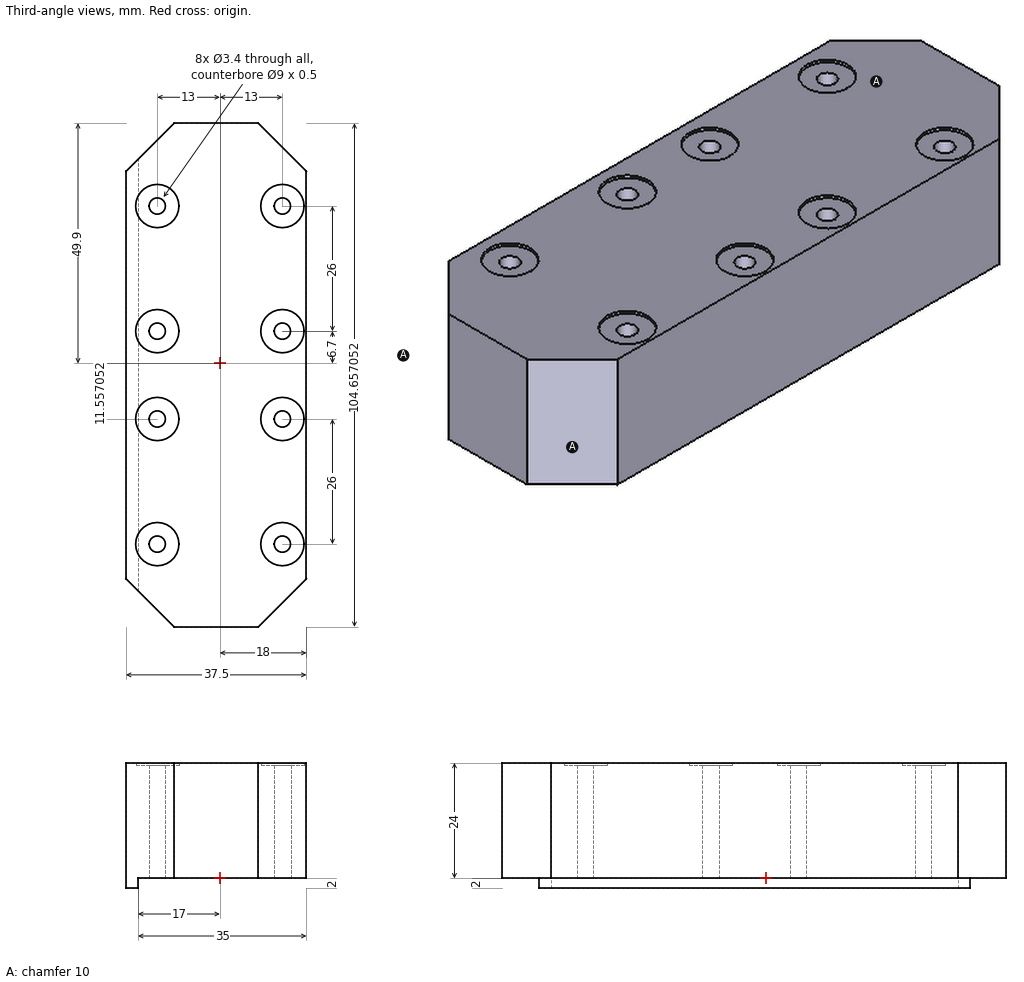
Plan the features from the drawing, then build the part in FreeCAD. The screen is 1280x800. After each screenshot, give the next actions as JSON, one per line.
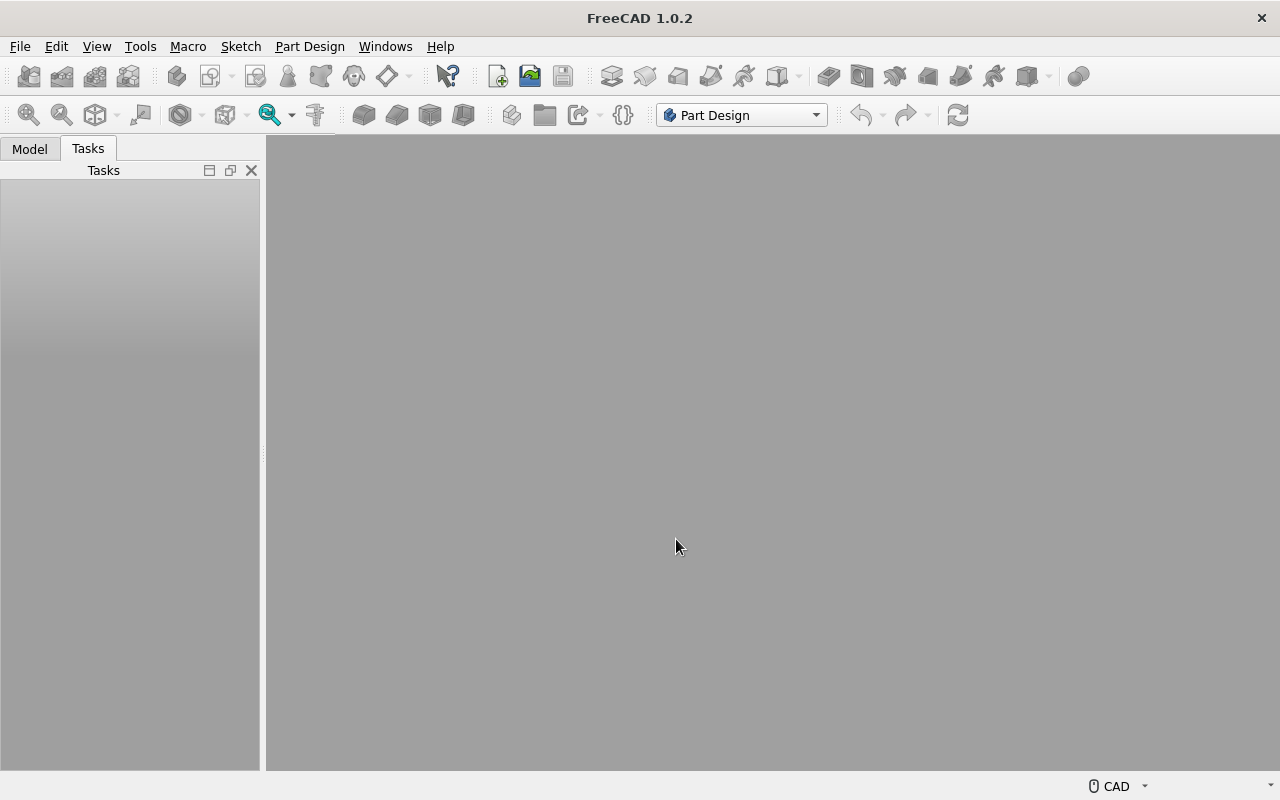
{"action": "left_click", "coordinate": [497, 76]}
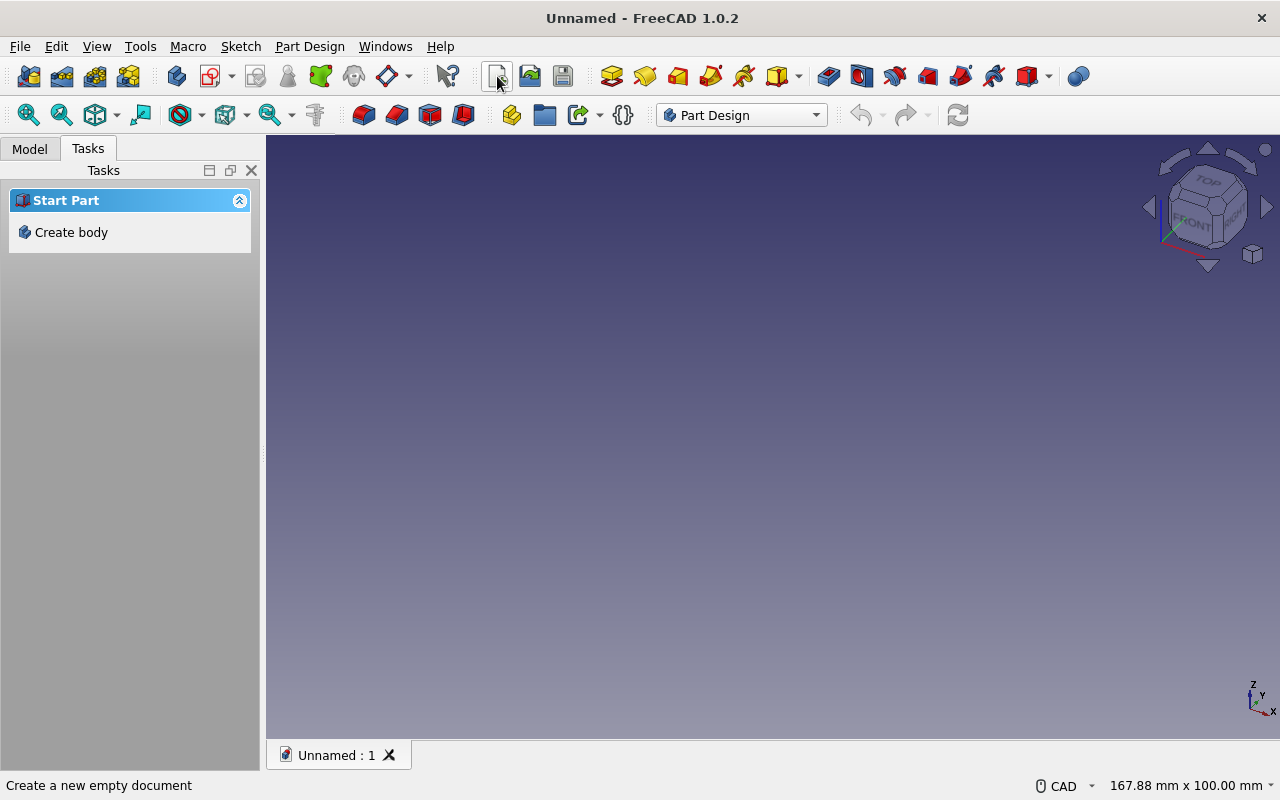
{"action": "left_click", "coordinate": [210, 76]}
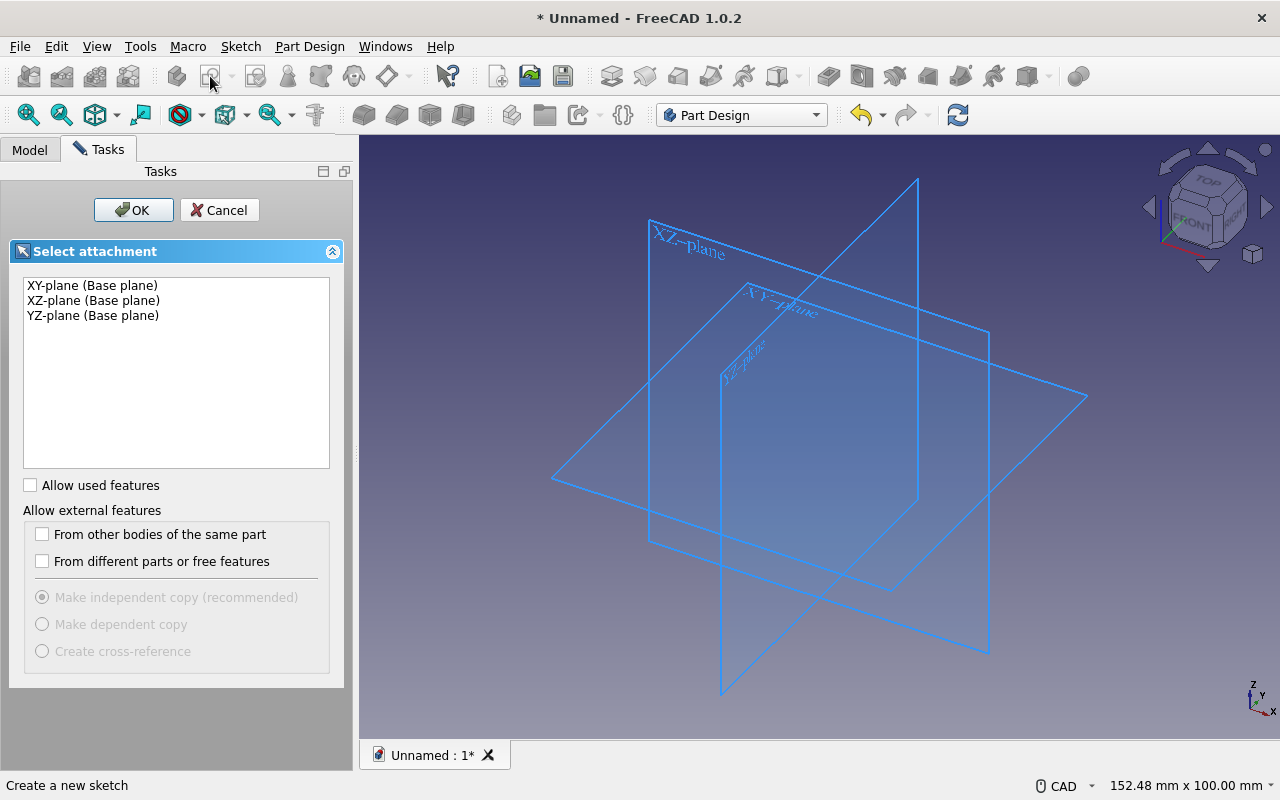
{"action": "left_click", "coordinate": [84, 286]}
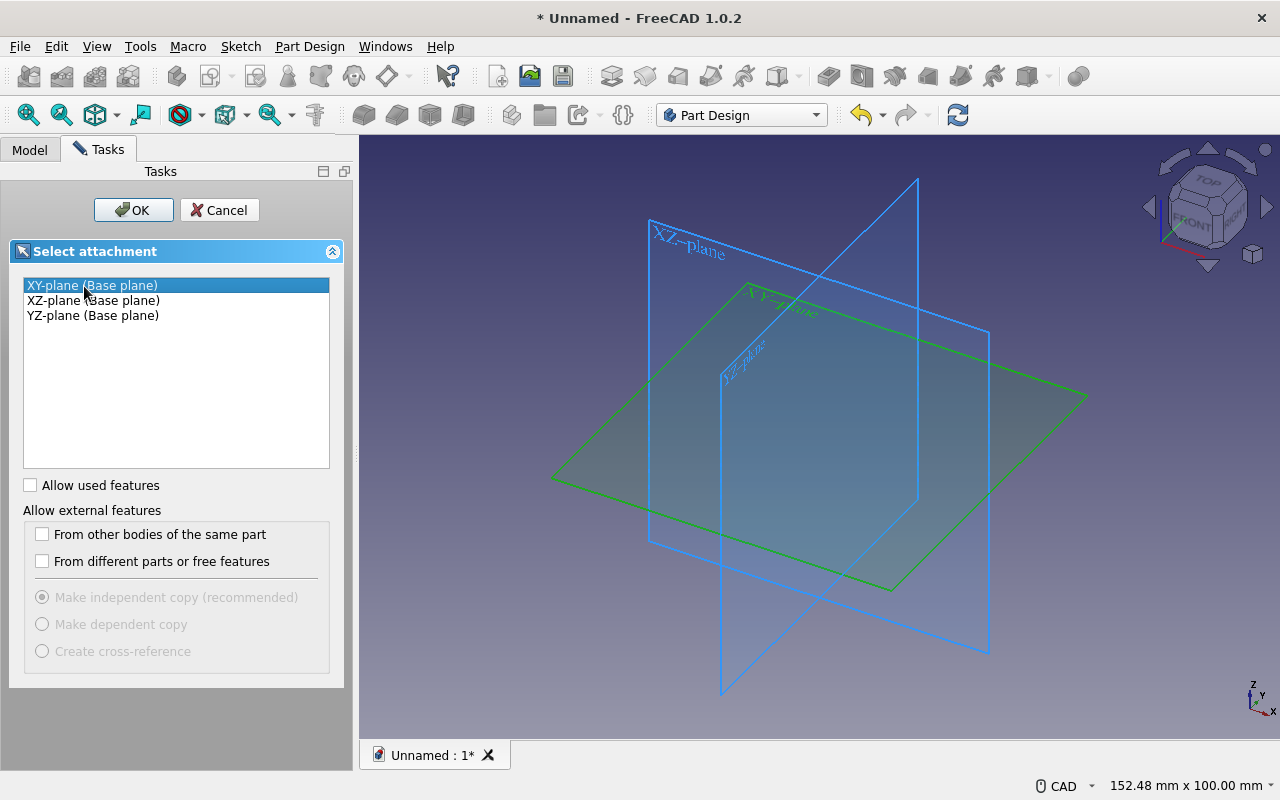
{"action": "left_click", "coordinate": [134, 210]}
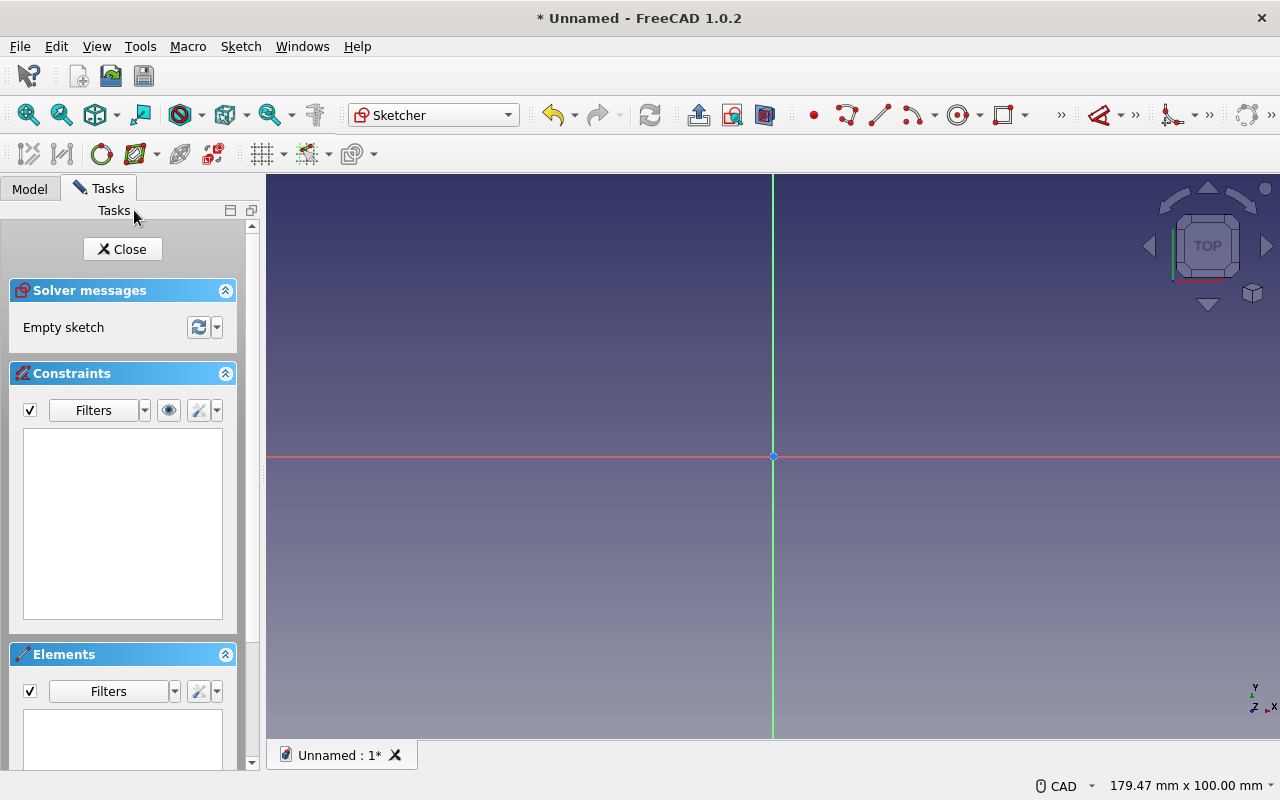
{"action": "scroll", "coordinate": [574, 429], "scroll_direction": "down", "scroll_amount": 2}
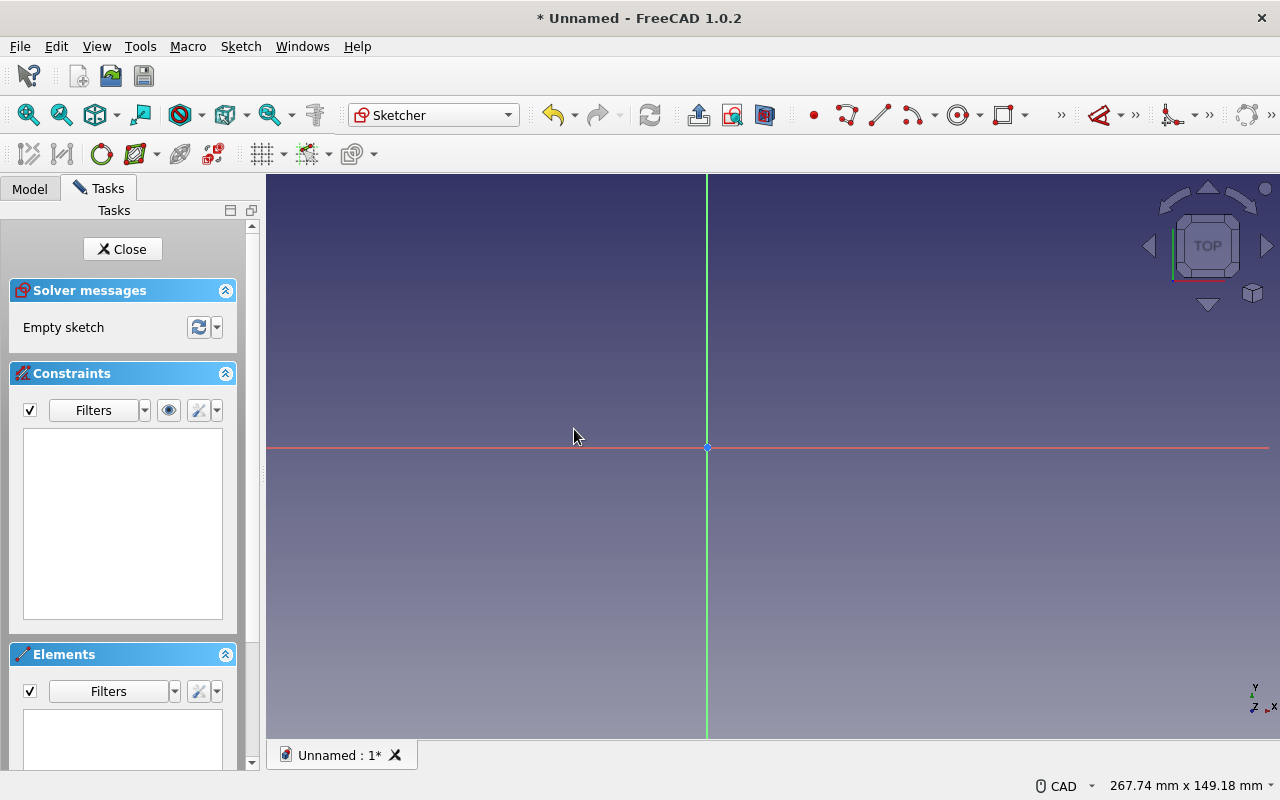
{"action": "left_click", "coordinate": [1002, 116]}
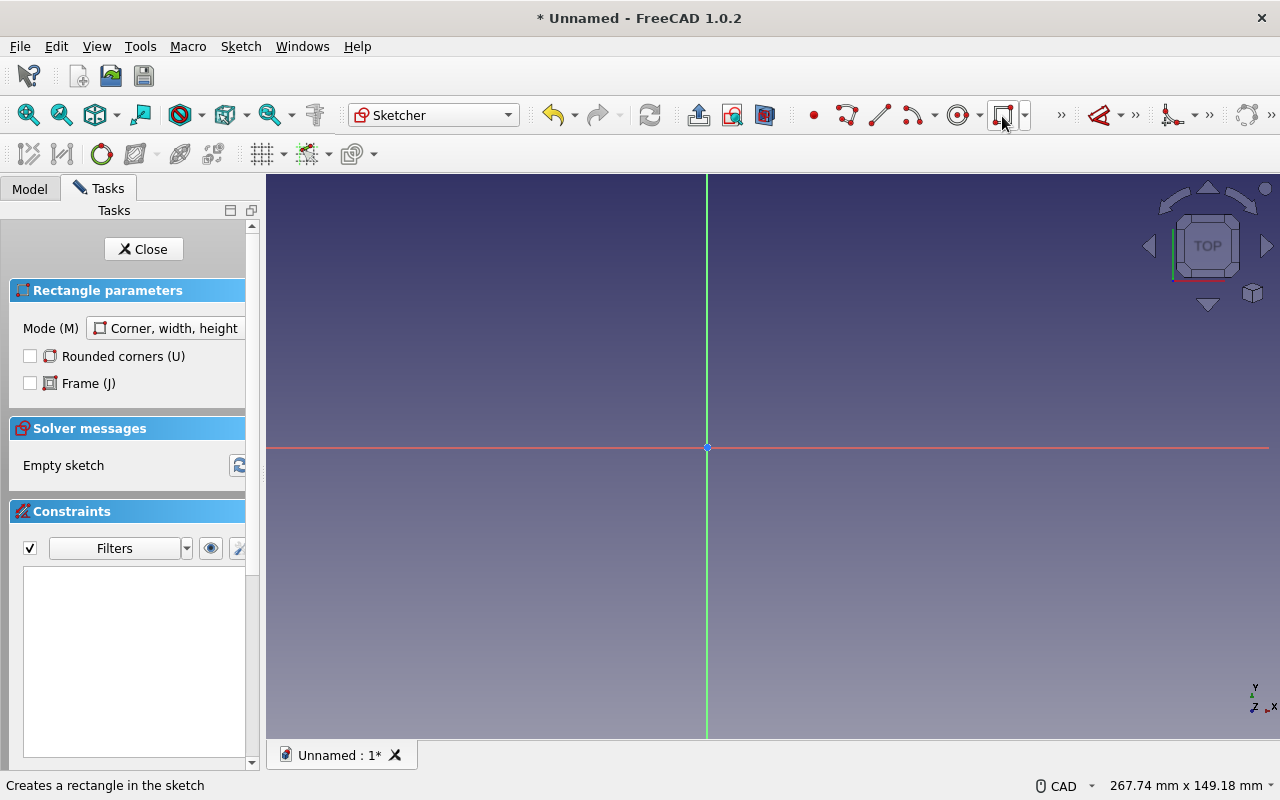
{"action": "left_click", "coordinate": [634, 259]}
{"action": "mouse_move", "coordinate": [776, 655]}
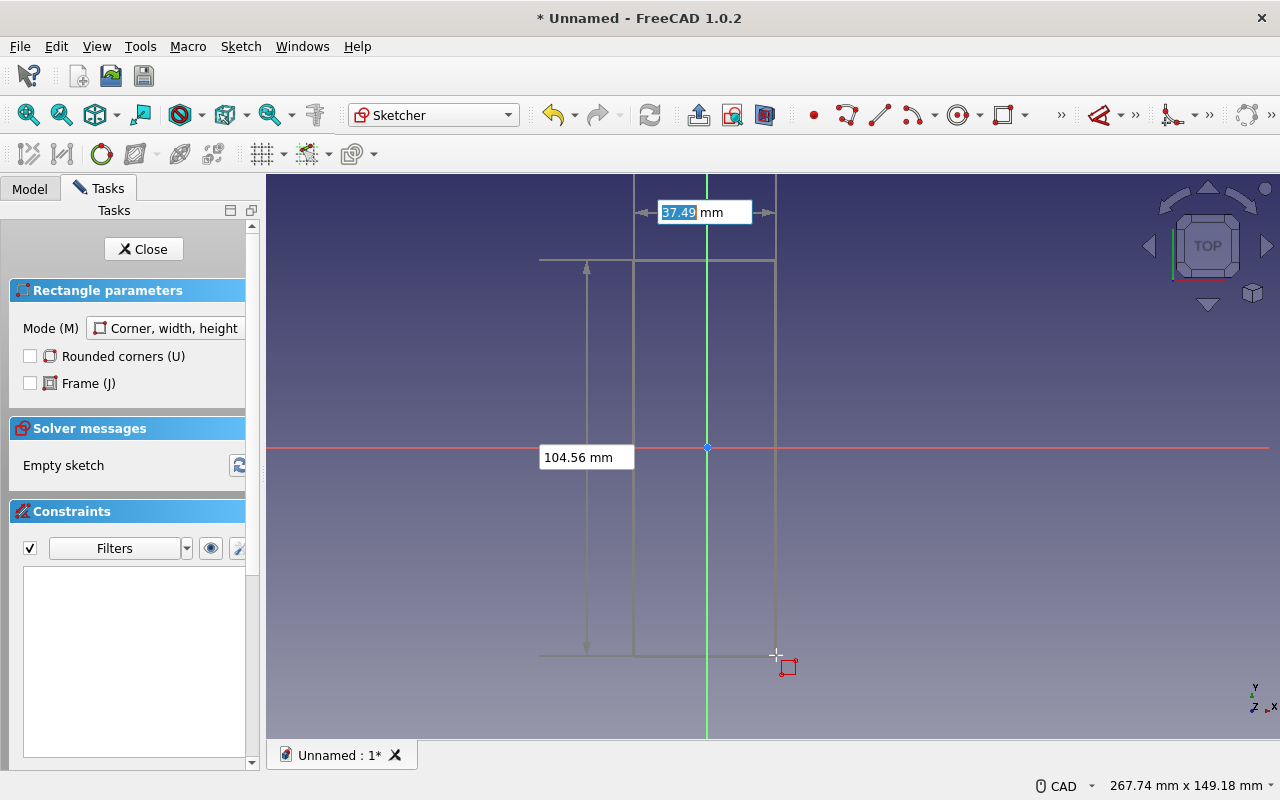
{"action": "type", "text": "37.5"}
{"action": "key", "text": "Tab"}
{"action": "type", "text": "104.657052"}
{"action": "key", "text": "Return"}
{"action": "key", "text": "Escape"}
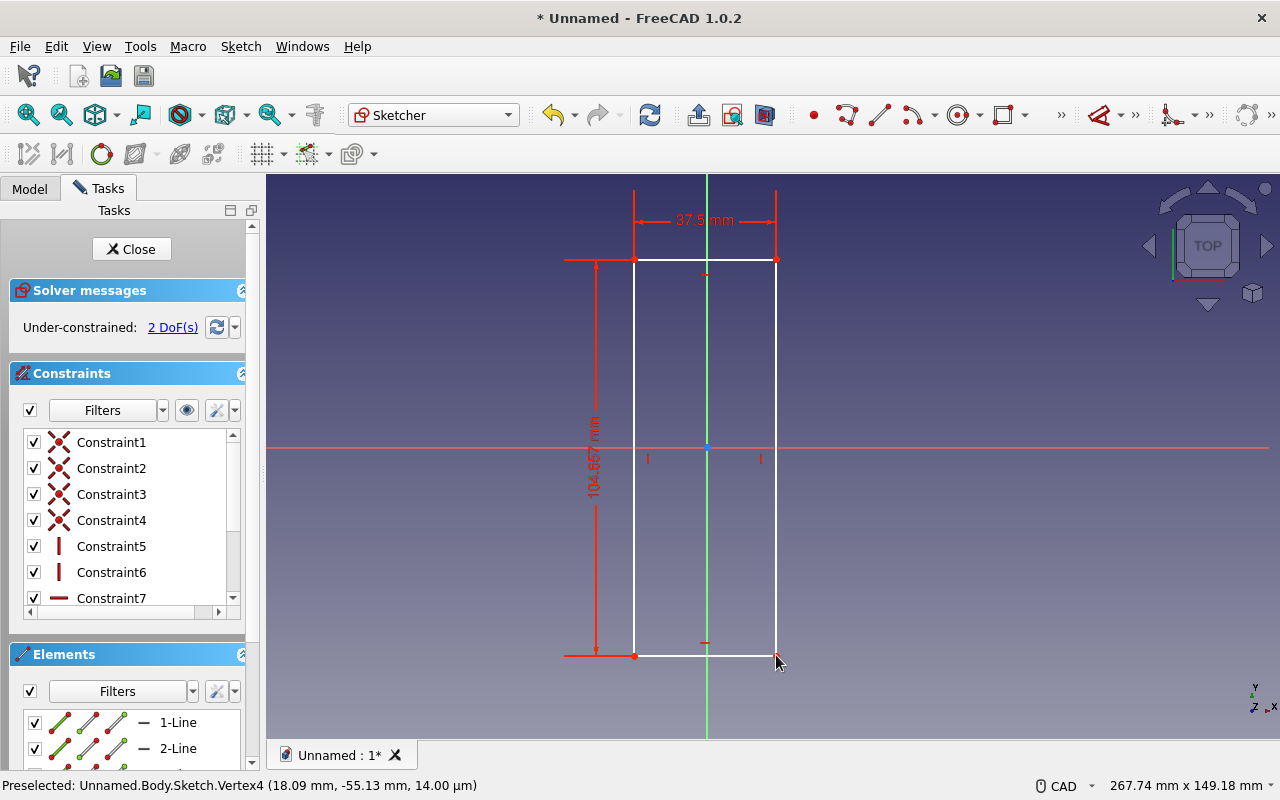
{"action": "left_click", "coordinate": [776, 656]}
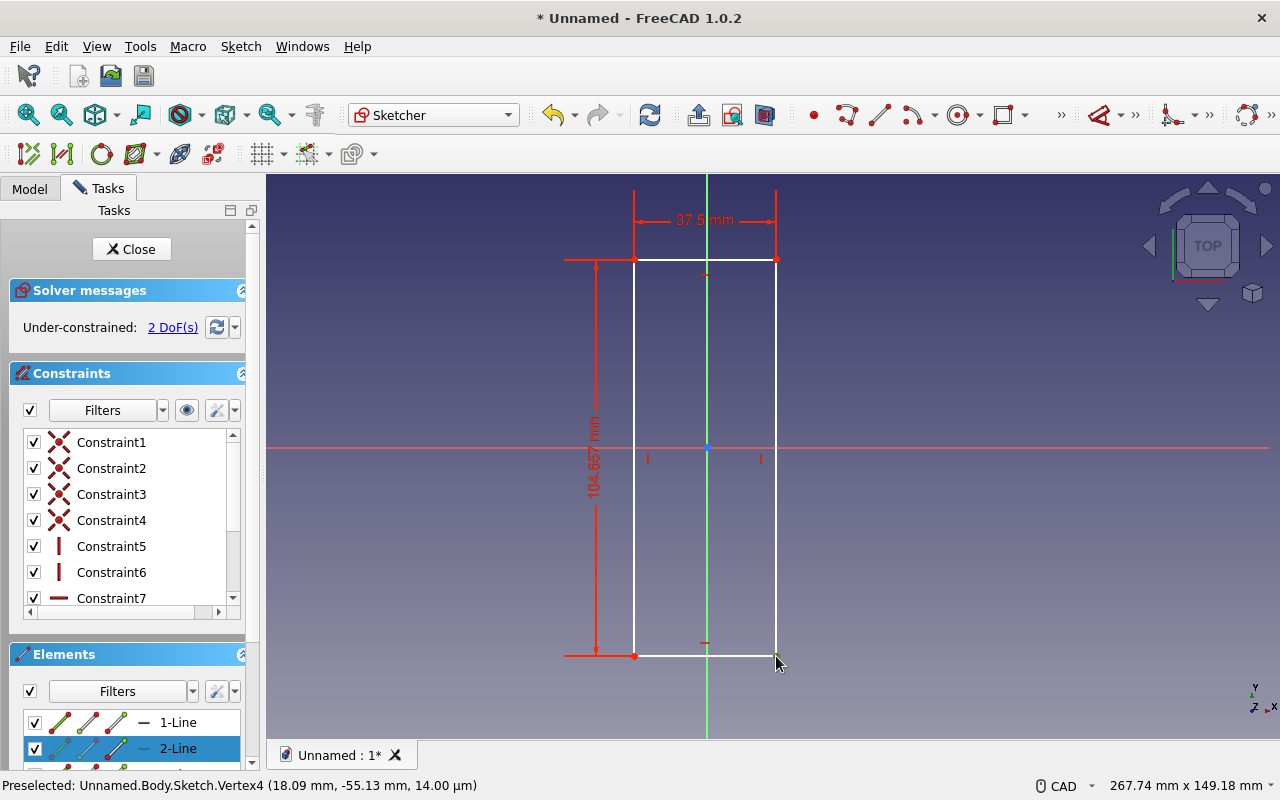
{"action": "left_click", "coordinate": [1120, 116]}